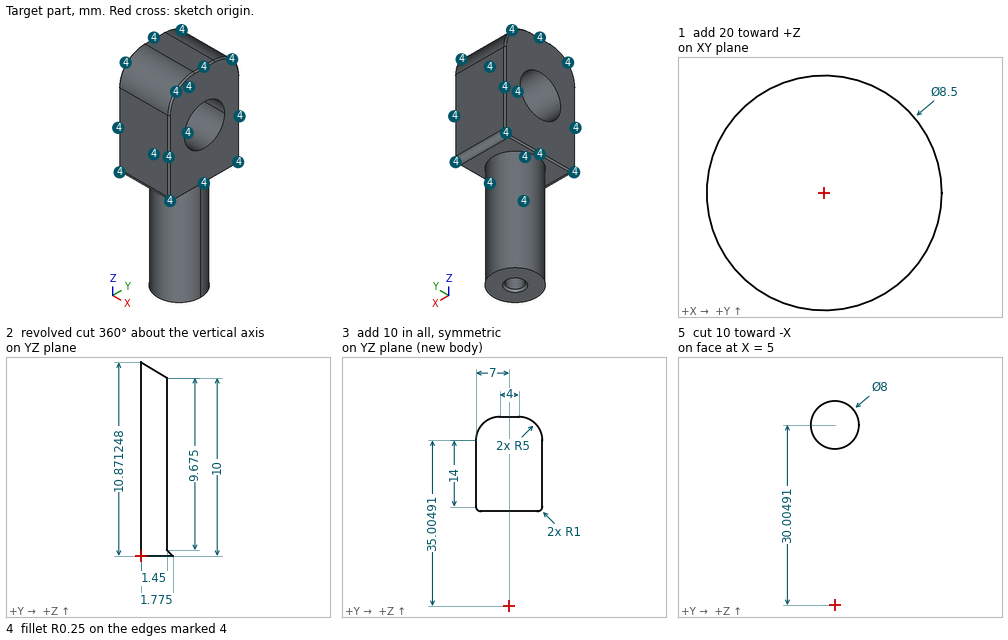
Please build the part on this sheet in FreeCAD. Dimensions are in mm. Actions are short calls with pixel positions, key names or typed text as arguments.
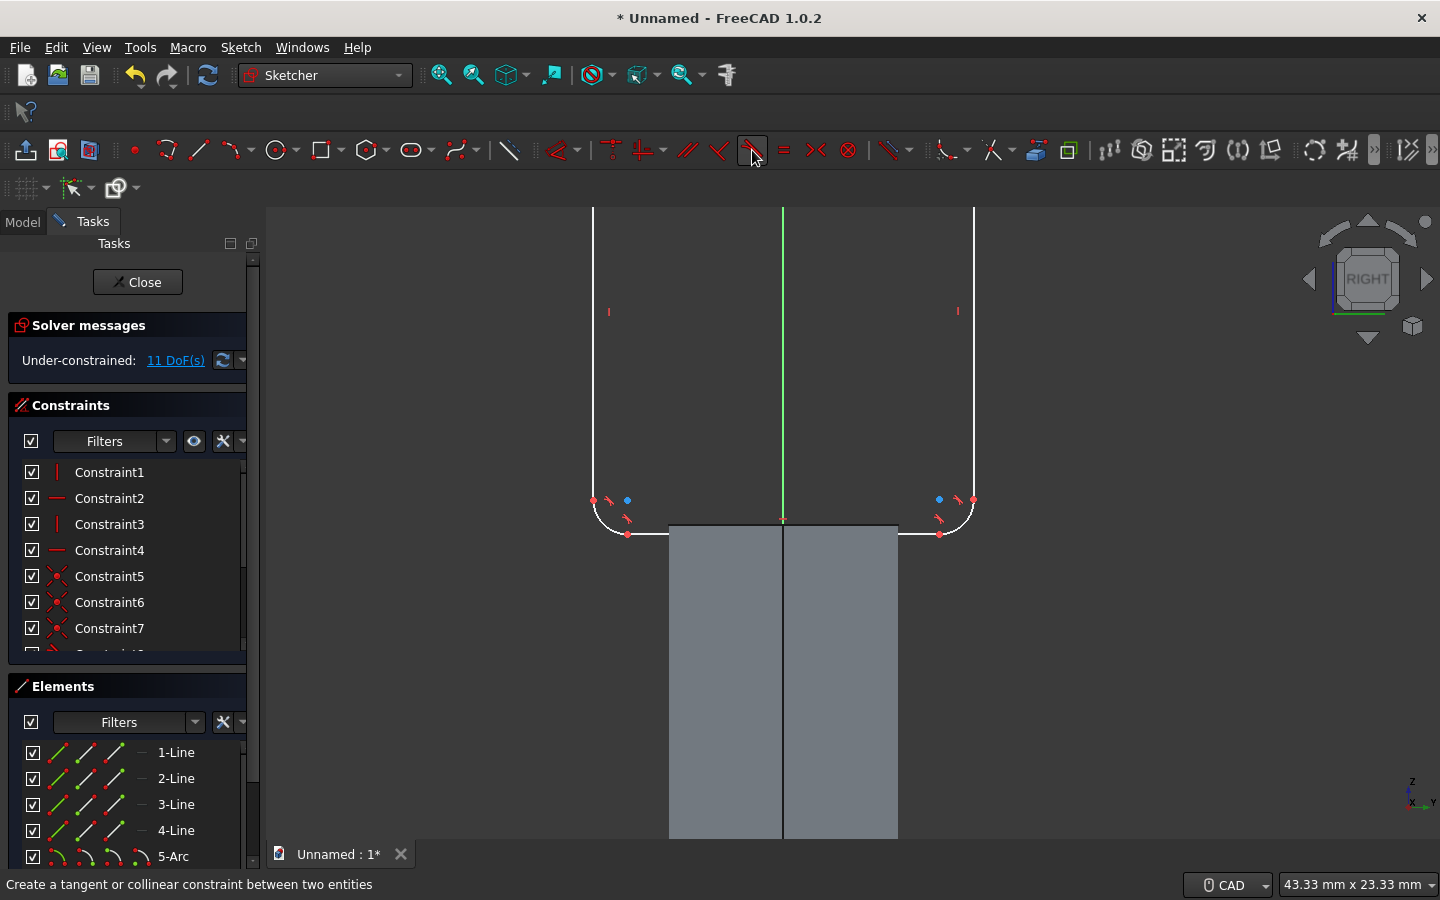
click(974, 386)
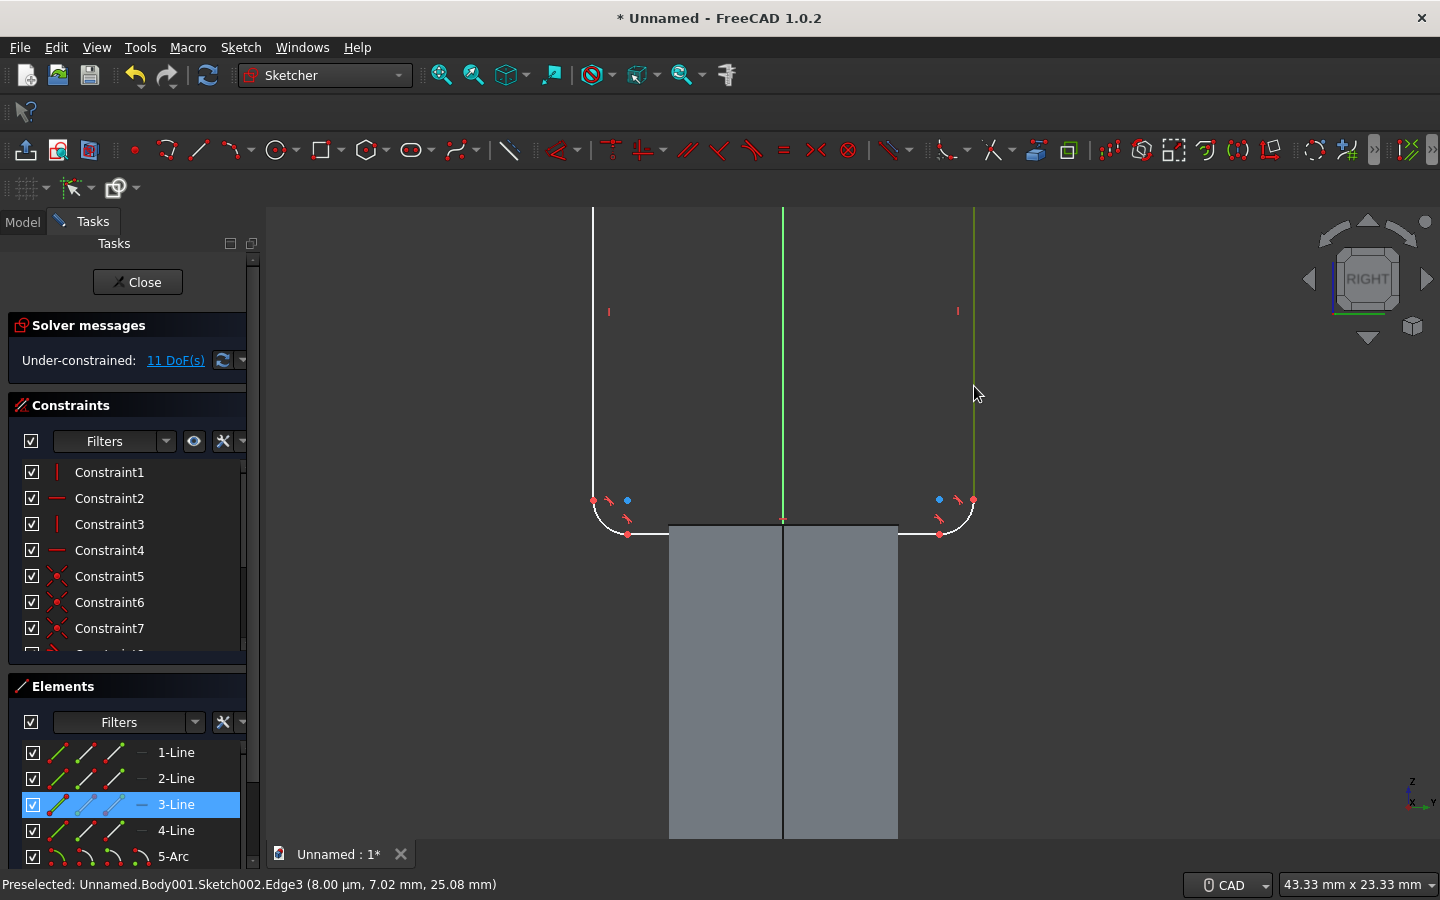
scroll(785, 522, down, 5)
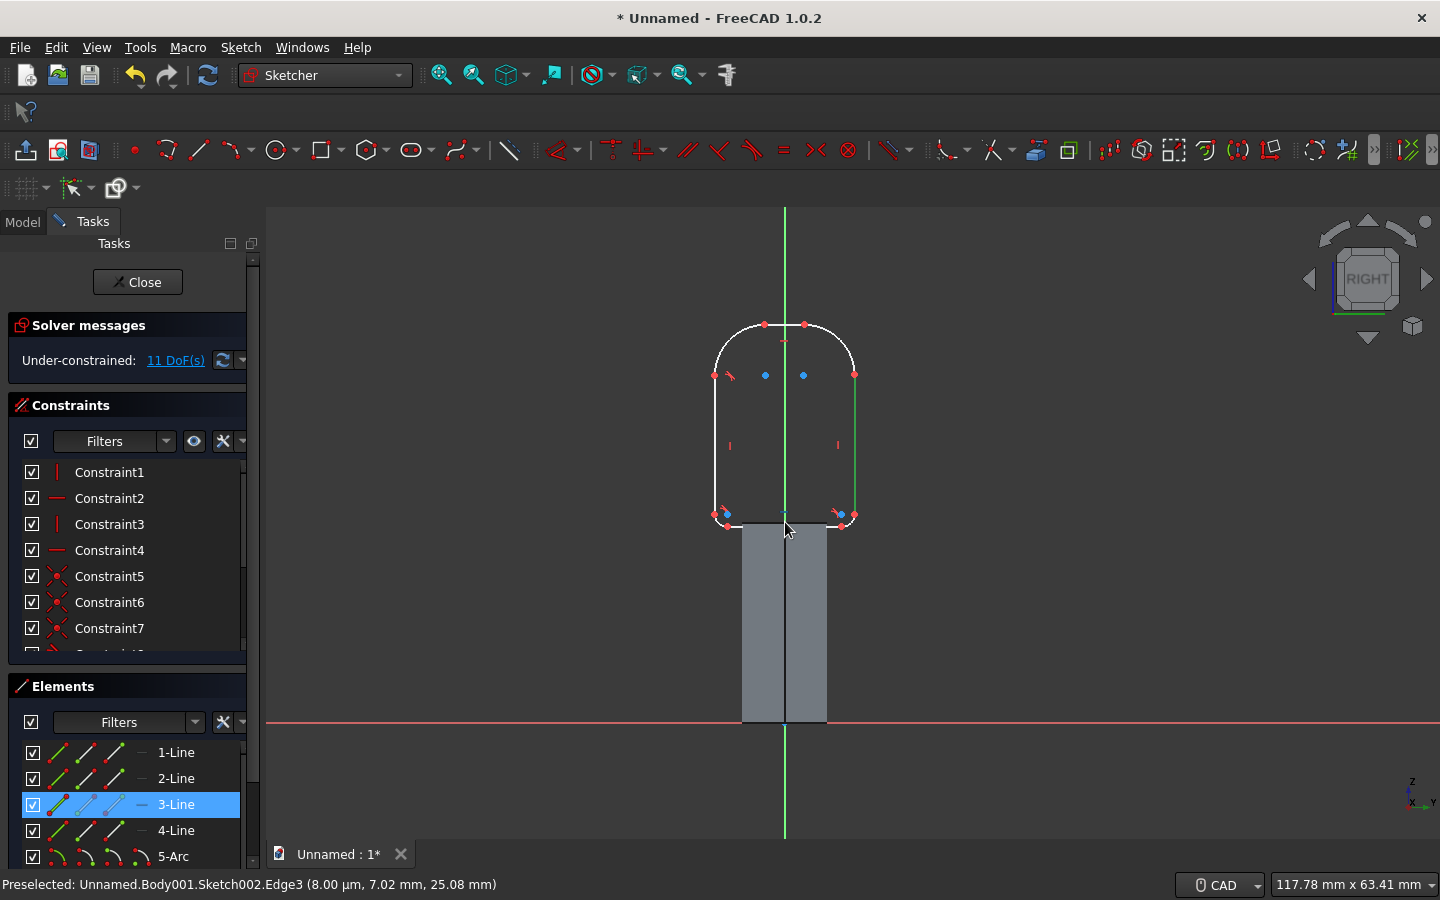
click(849, 352)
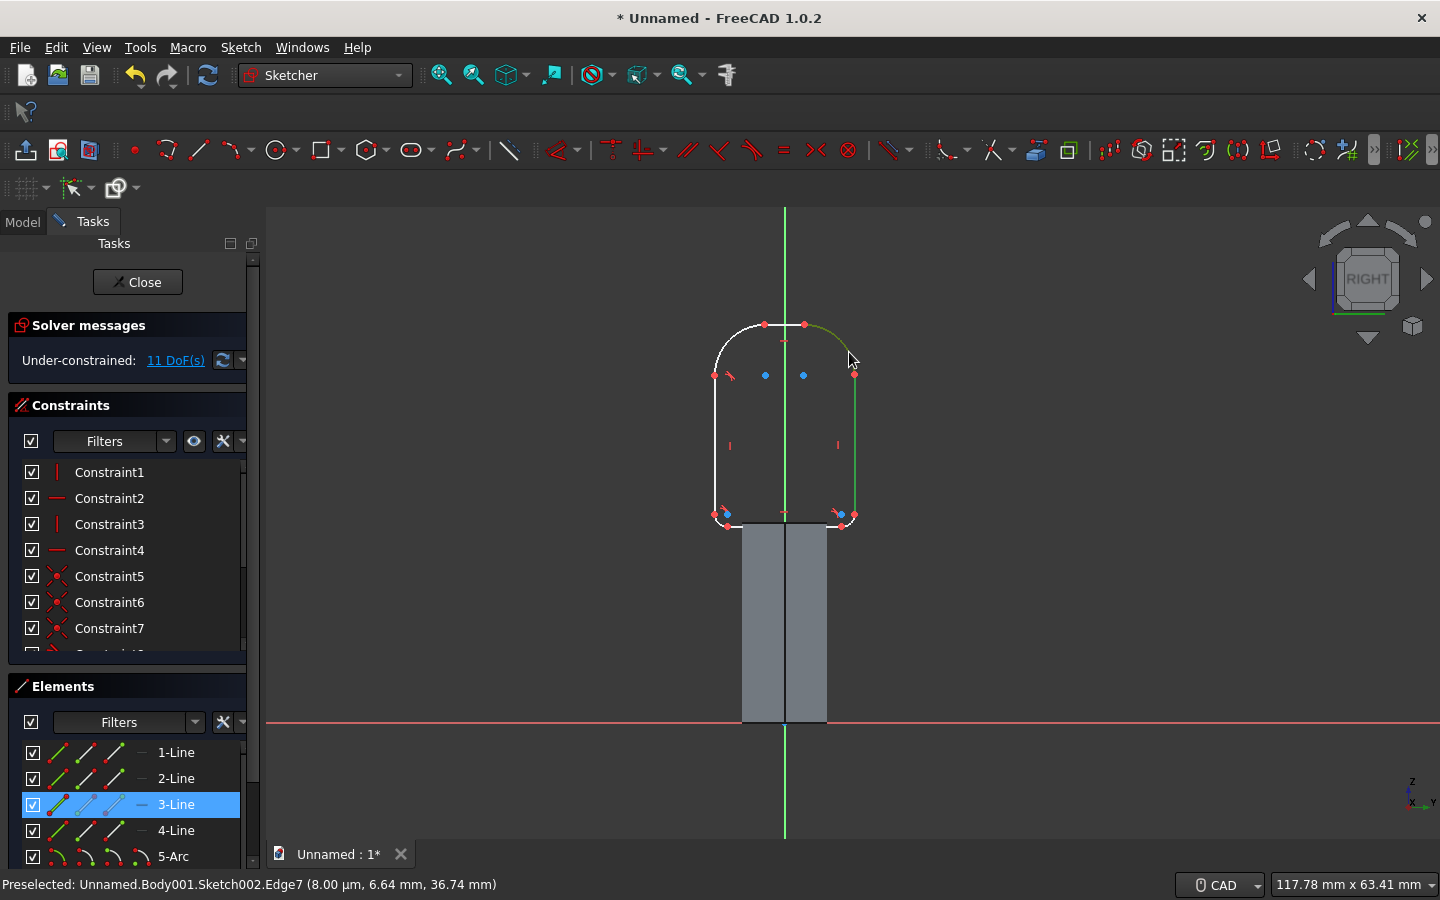
key(t)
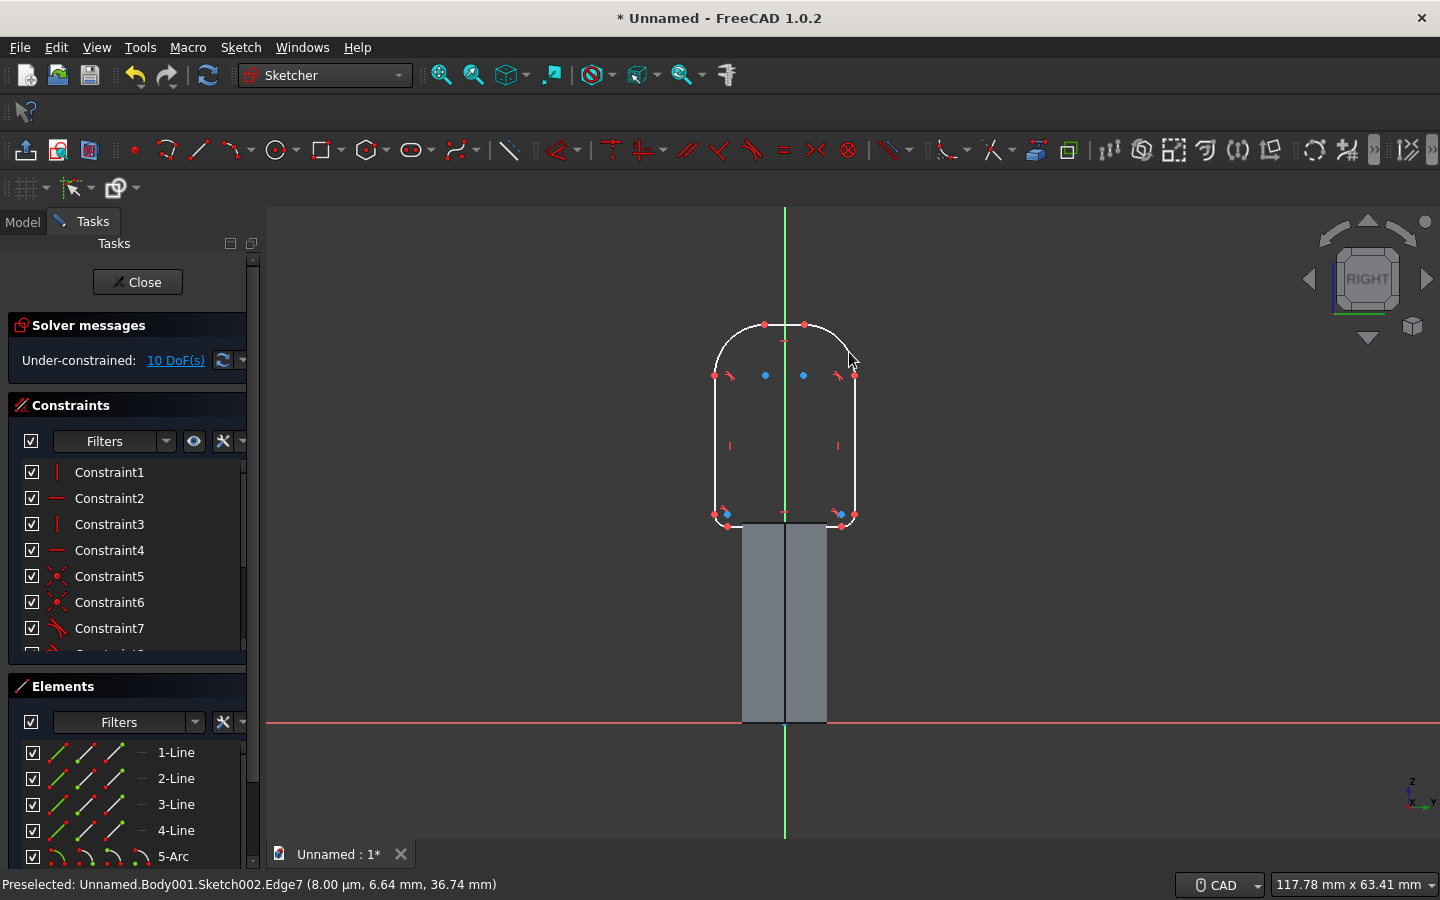
click(781, 325)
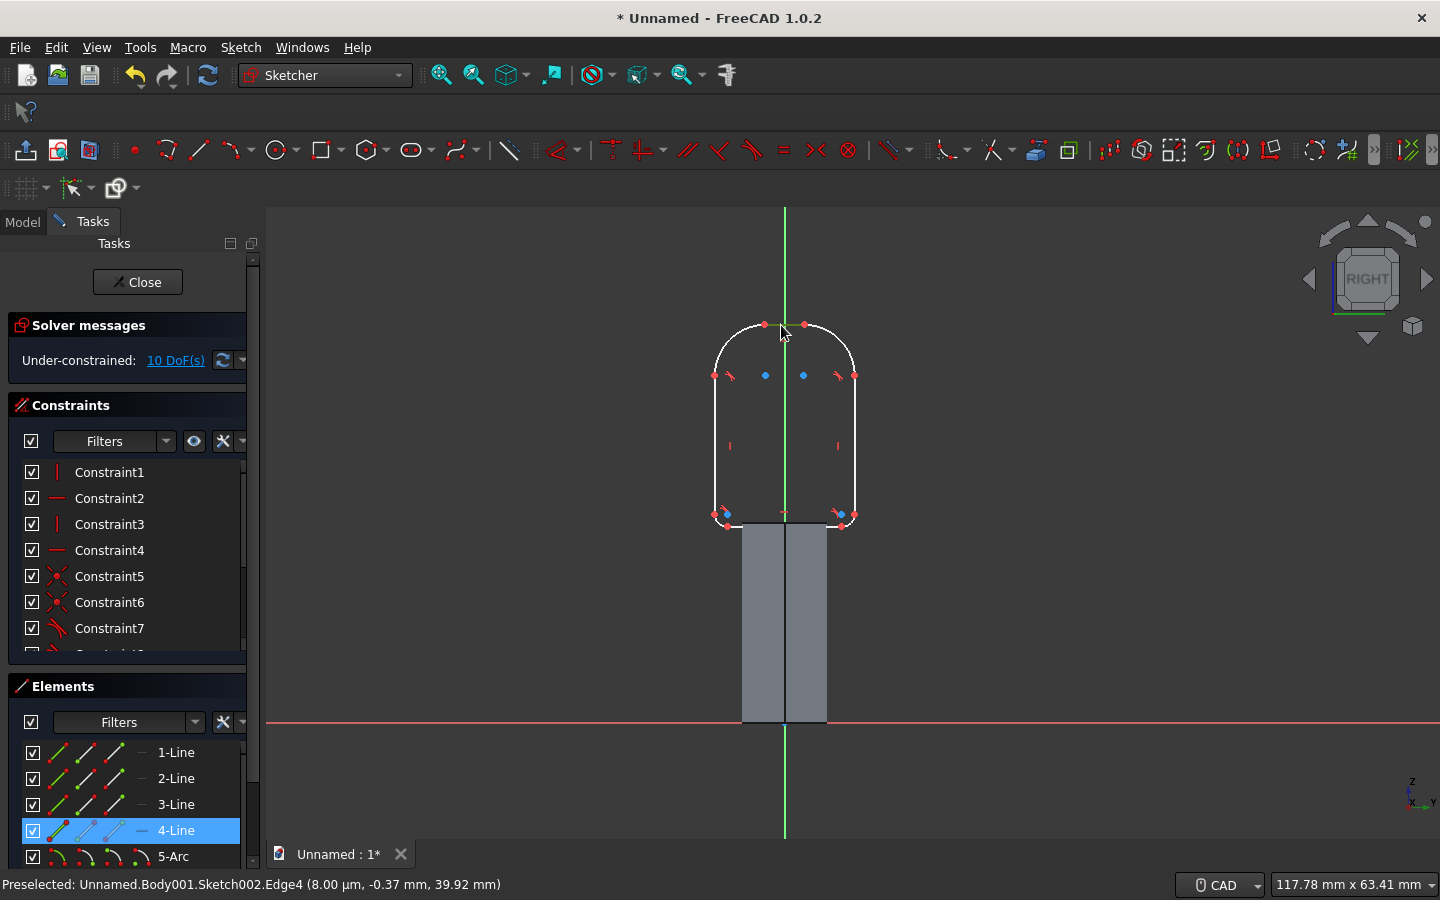
click(849, 353)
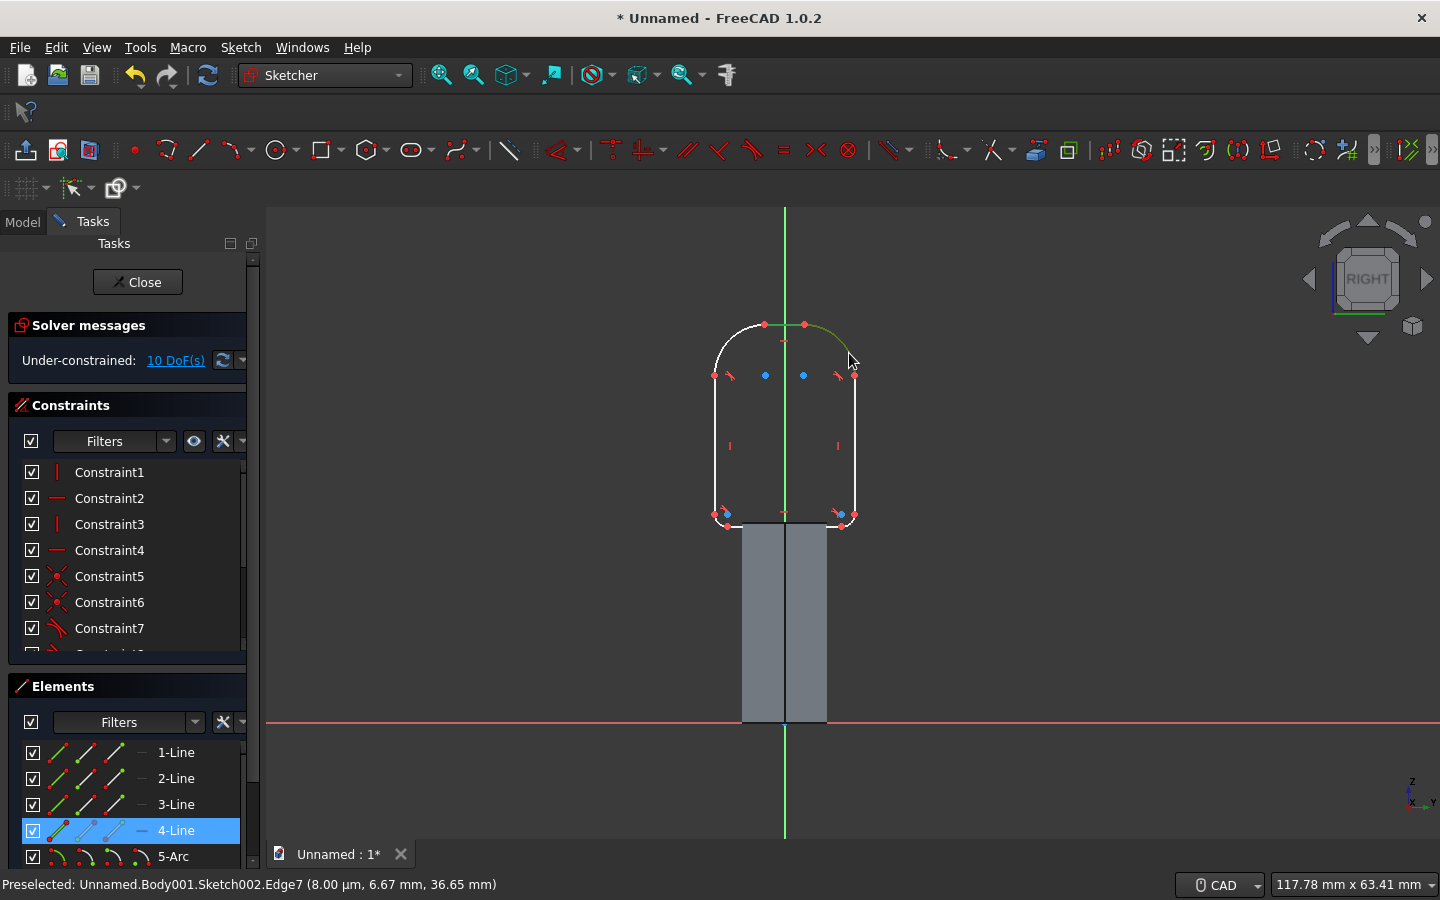
click(752, 150)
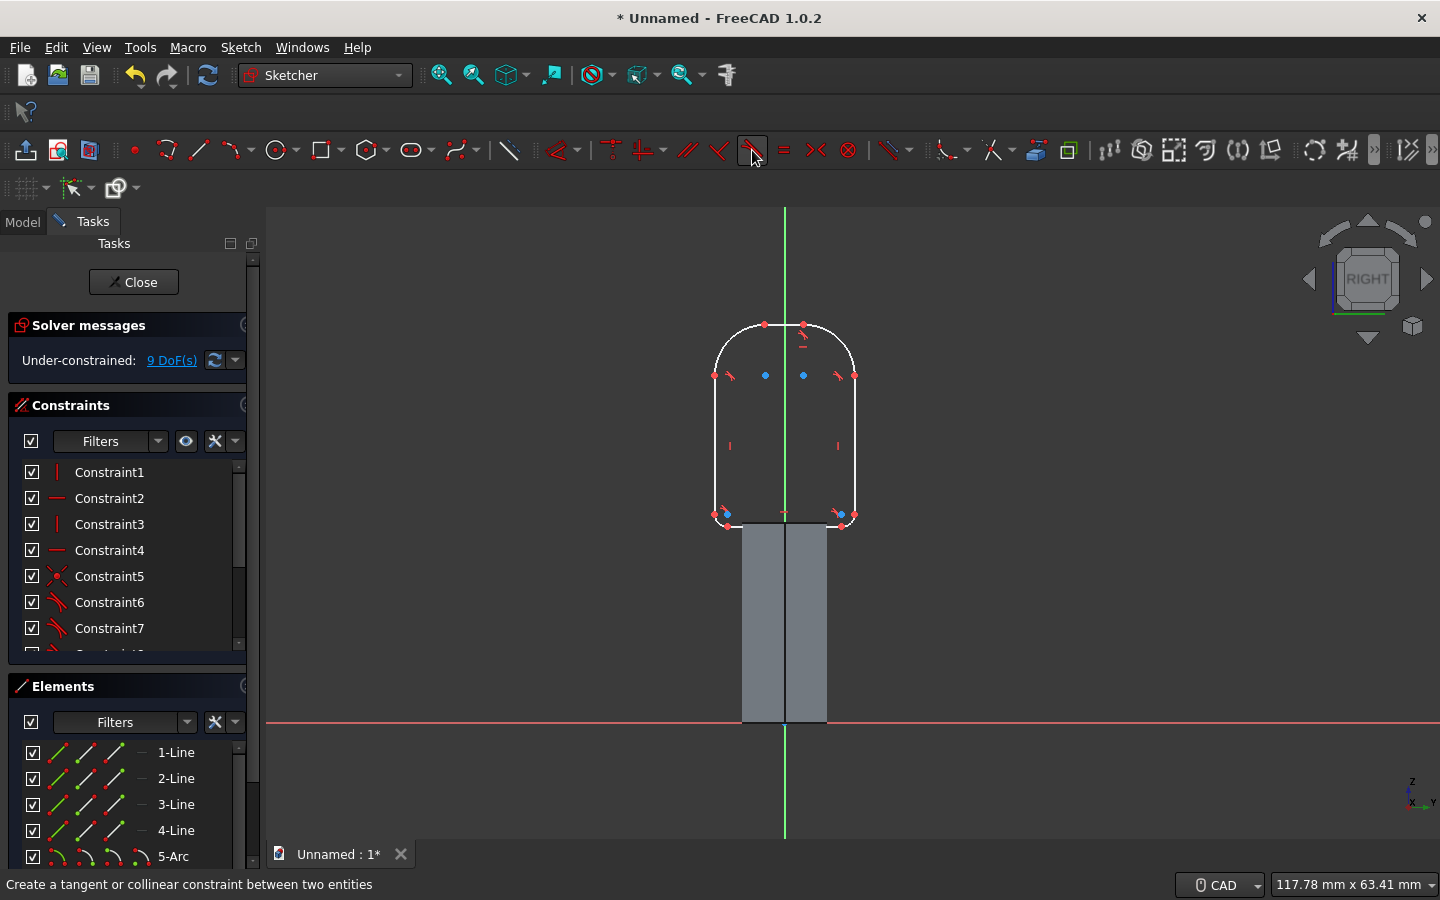
click(788, 325)